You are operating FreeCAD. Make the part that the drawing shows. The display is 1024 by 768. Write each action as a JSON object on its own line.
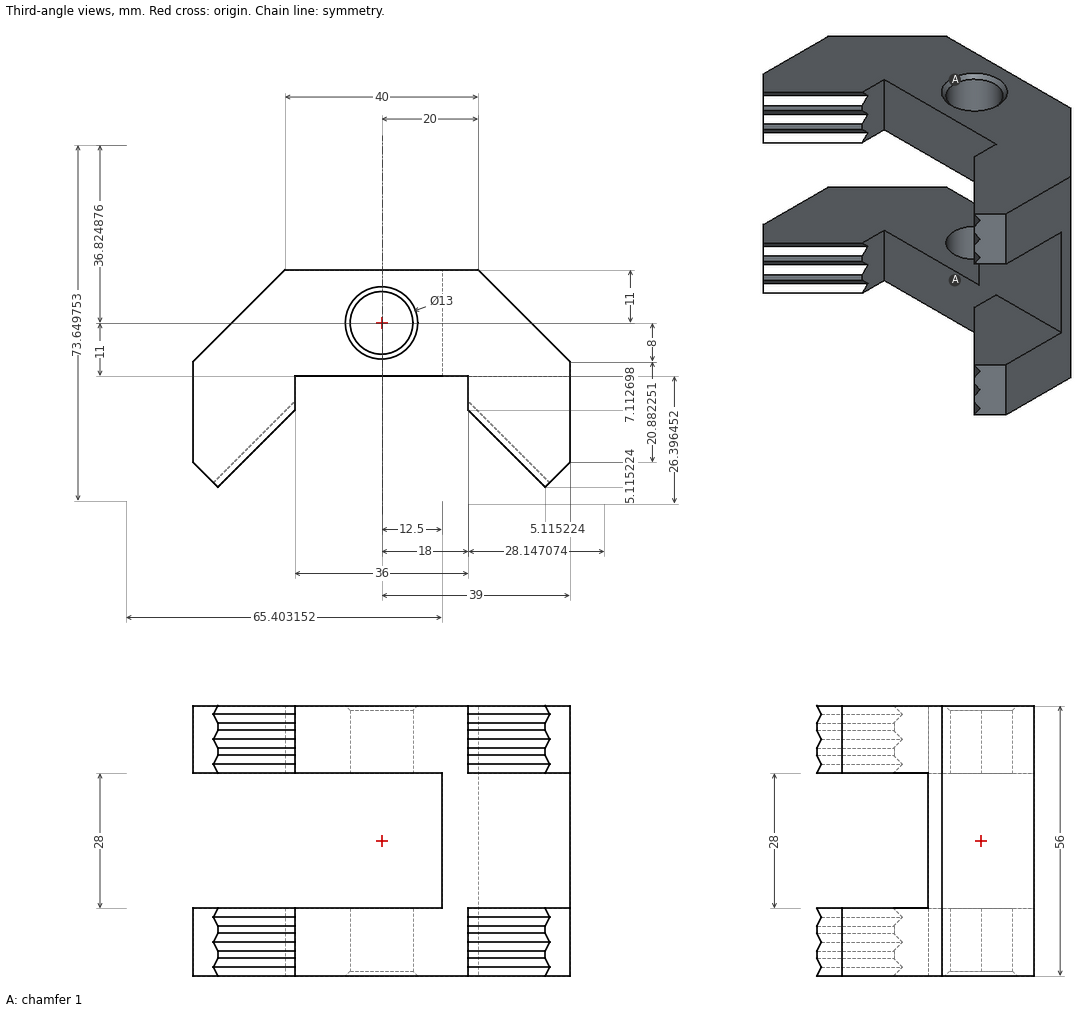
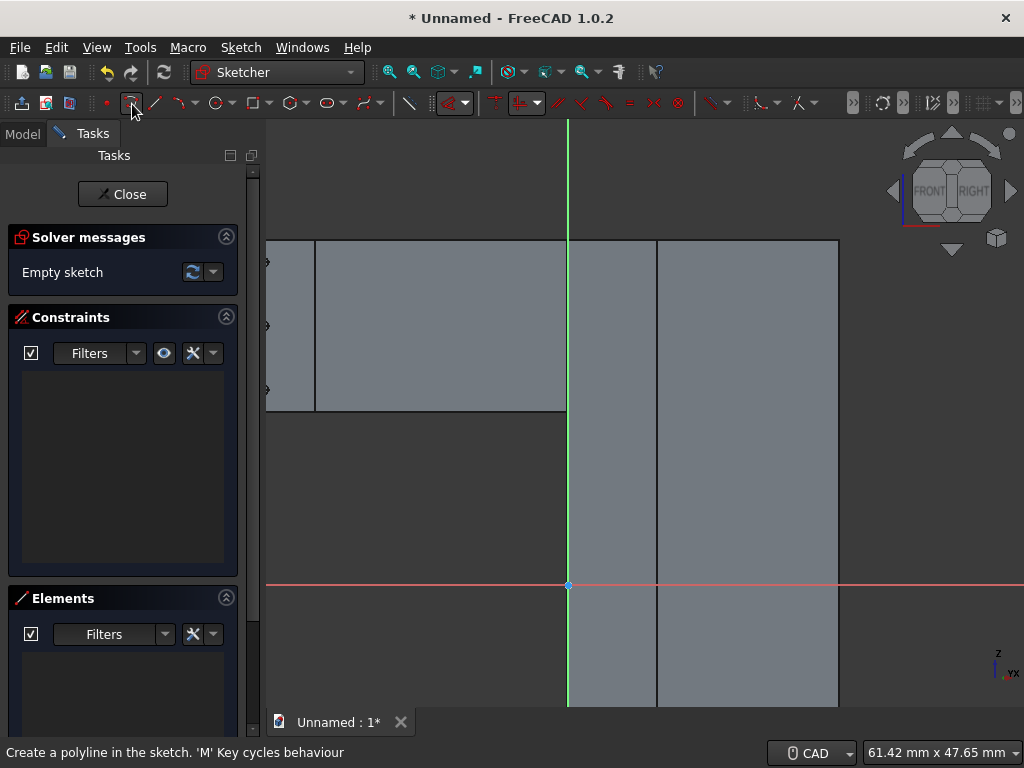
{"action": "scroll", "coordinate": [567, 349], "scroll_direction": "up", "scroll_amount": 14}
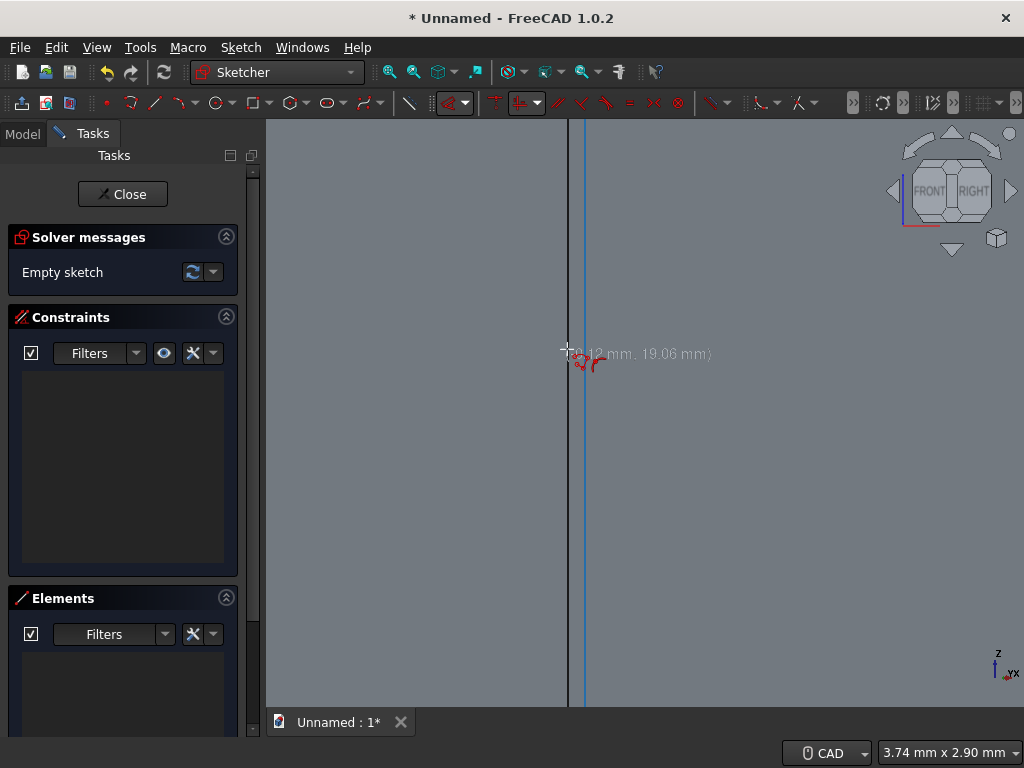
{"action": "left_click", "coordinate": [568, 338]}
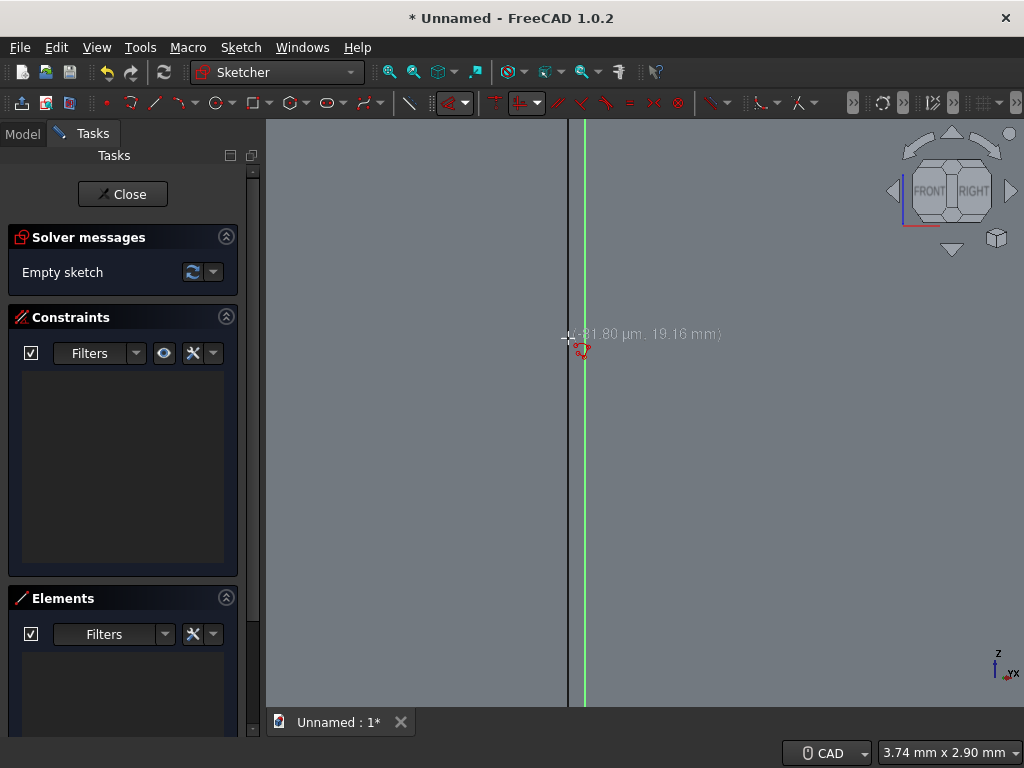
{"action": "scroll", "coordinate": [569, 350], "scroll_direction": "down", "scroll_amount": 14}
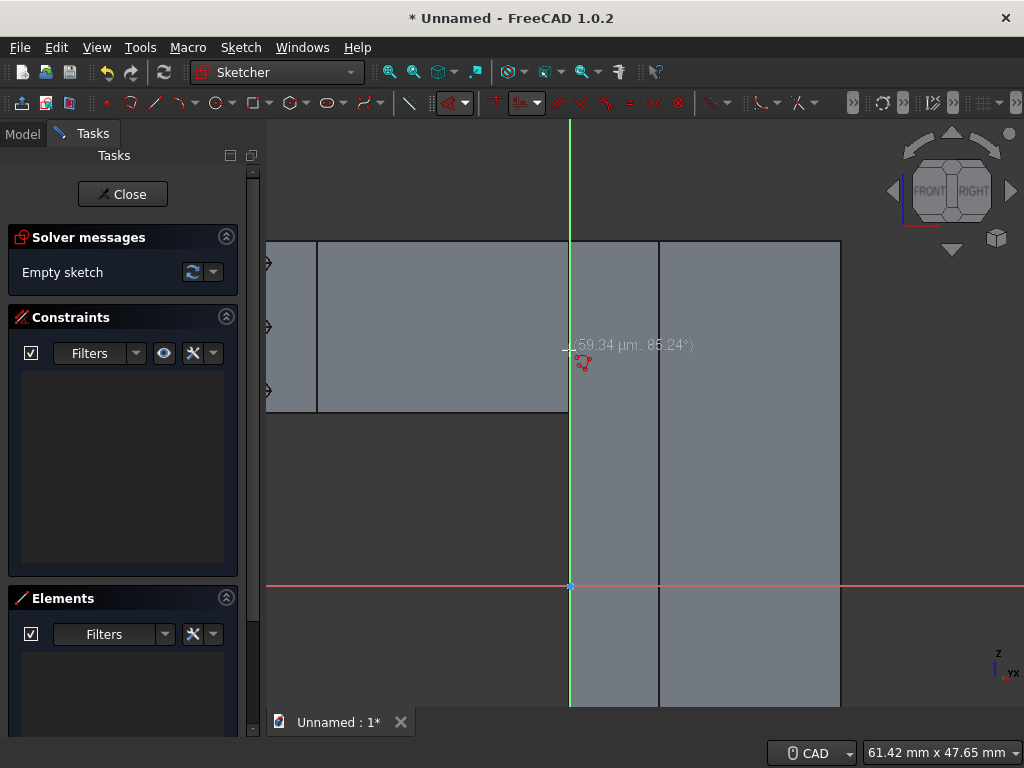
{"action": "left_click", "coordinate": [585, 327]}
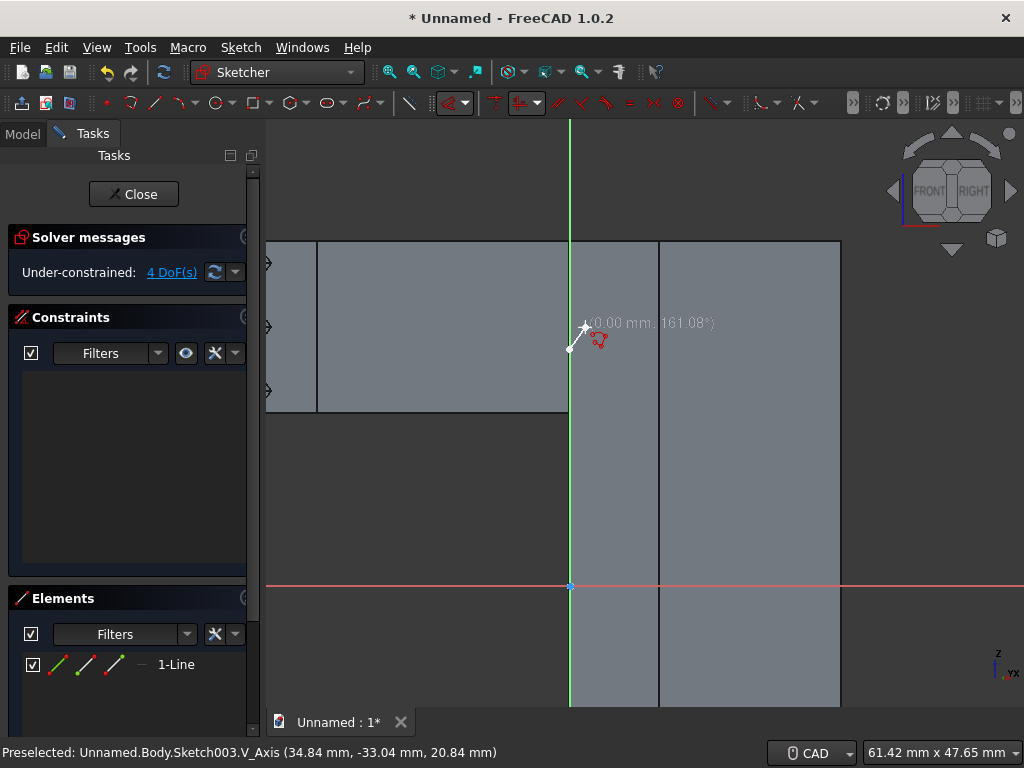
{"action": "scroll", "coordinate": [569, 304], "scroll_direction": "up", "scroll_amount": 14}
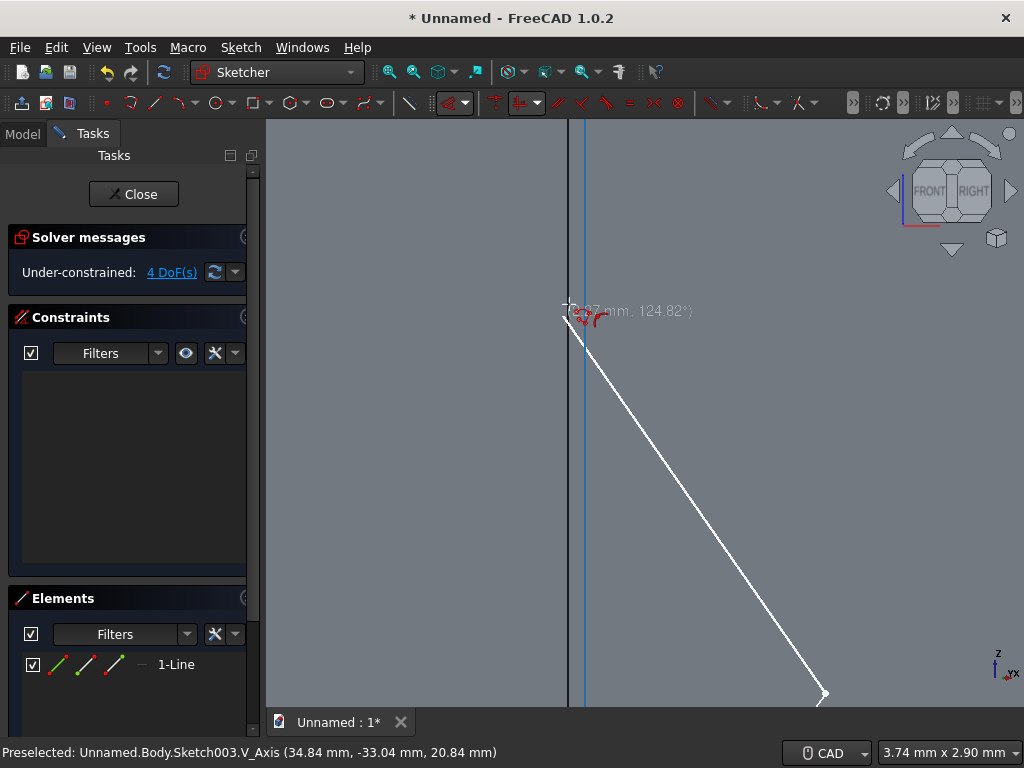
{"action": "left_click", "coordinate": [568, 305]}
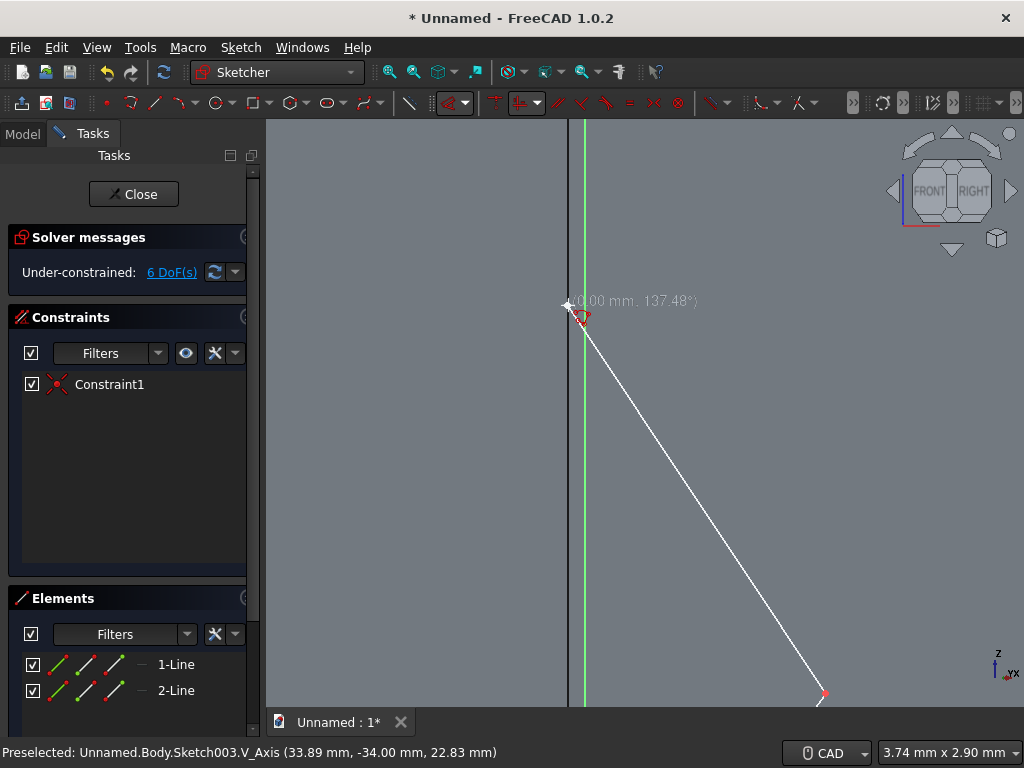
{"action": "scroll", "coordinate": [569, 304], "scroll_direction": "down", "scroll_amount": 14}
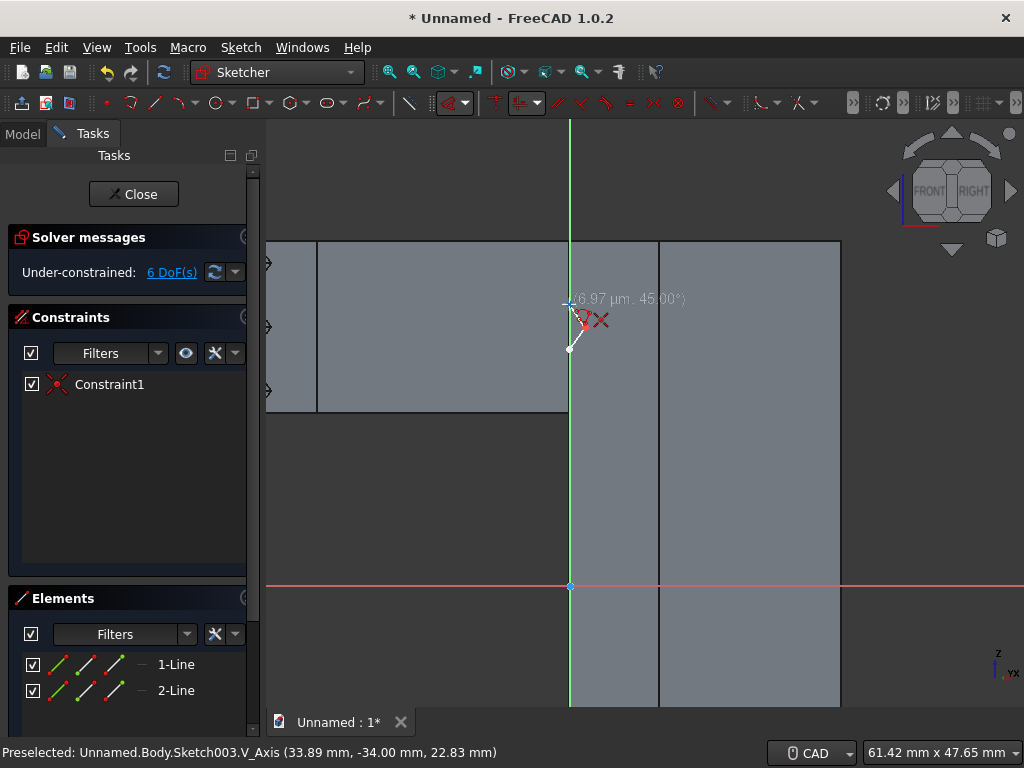
{"action": "scroll", "coordinate": [569, 350], "scroll_direction": "up", "scroll_amount": 14}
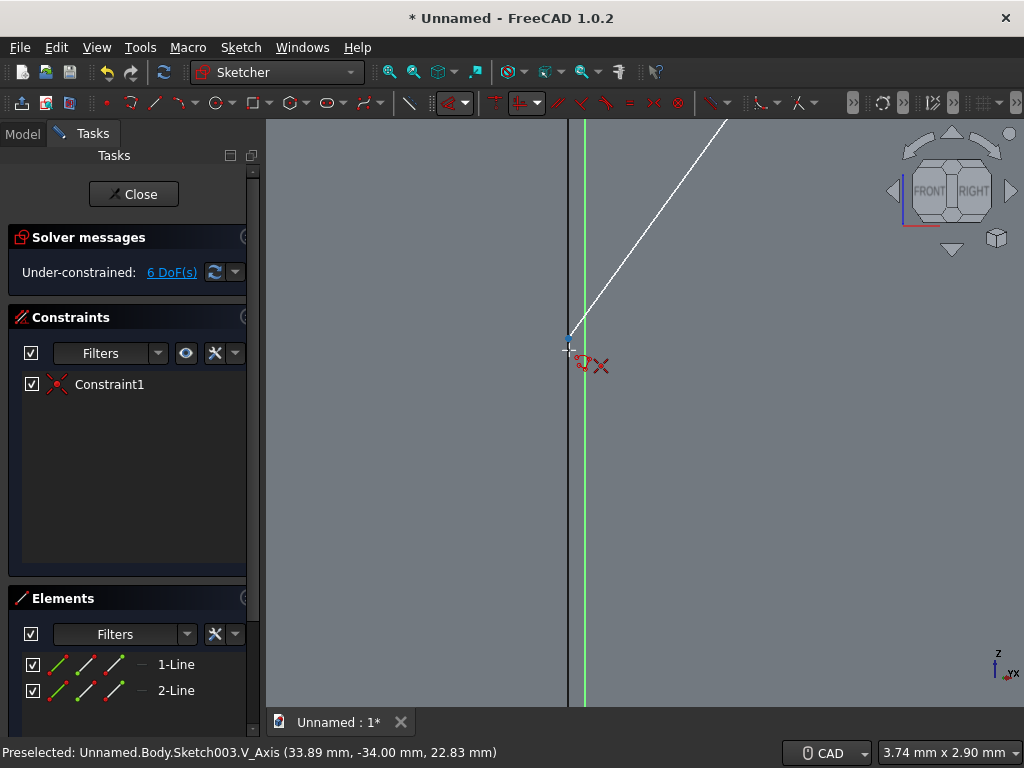
{"action": "left_click", "coordinate": [568, 339]}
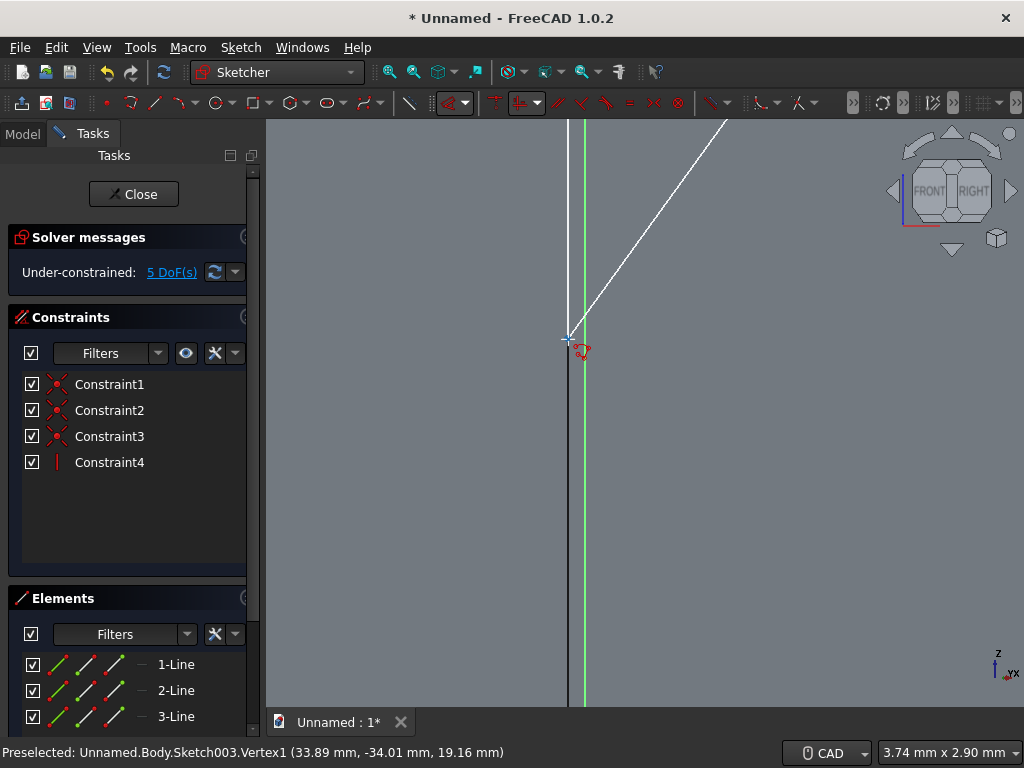
{"action": "scroll", "coordinate": [569, 350], "scroll_direction": "down", "scroll_amount": 14}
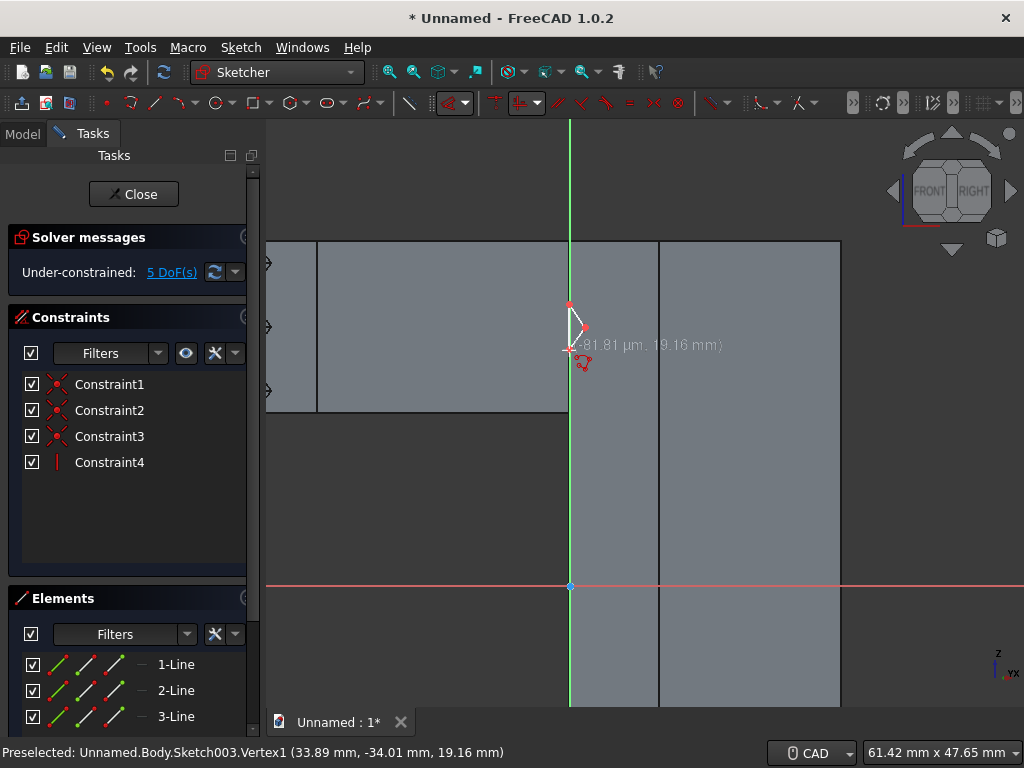
{"action": "scroll", "coordinate": [569, 413], "scroll_direction": "up", "scroll_amount": 14}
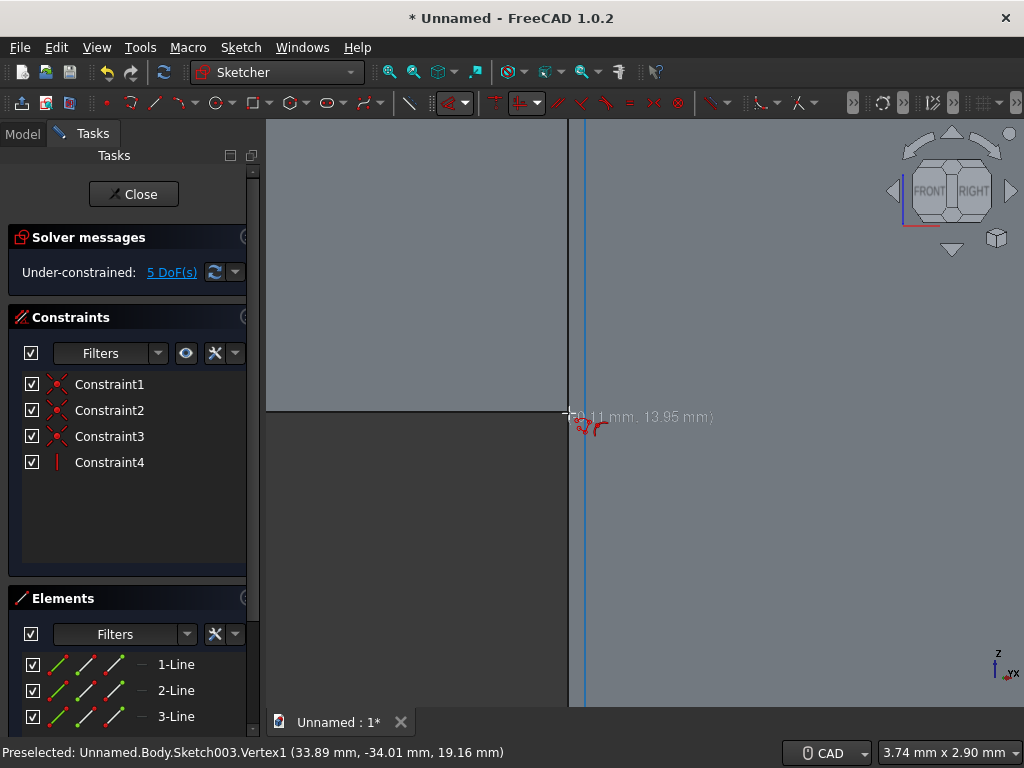
{"action": "left_click", "coordinate": [568, 412]}